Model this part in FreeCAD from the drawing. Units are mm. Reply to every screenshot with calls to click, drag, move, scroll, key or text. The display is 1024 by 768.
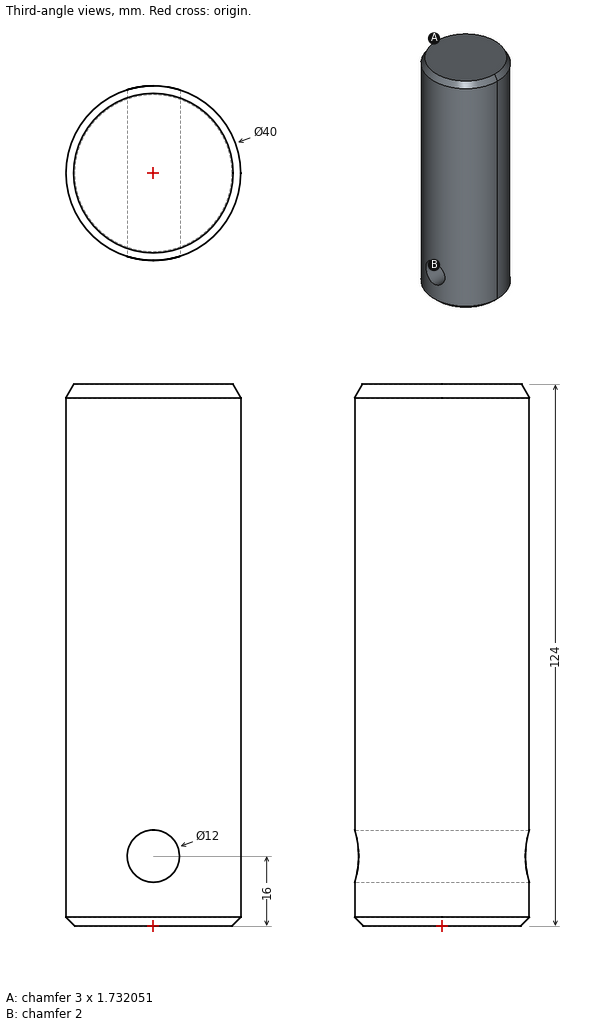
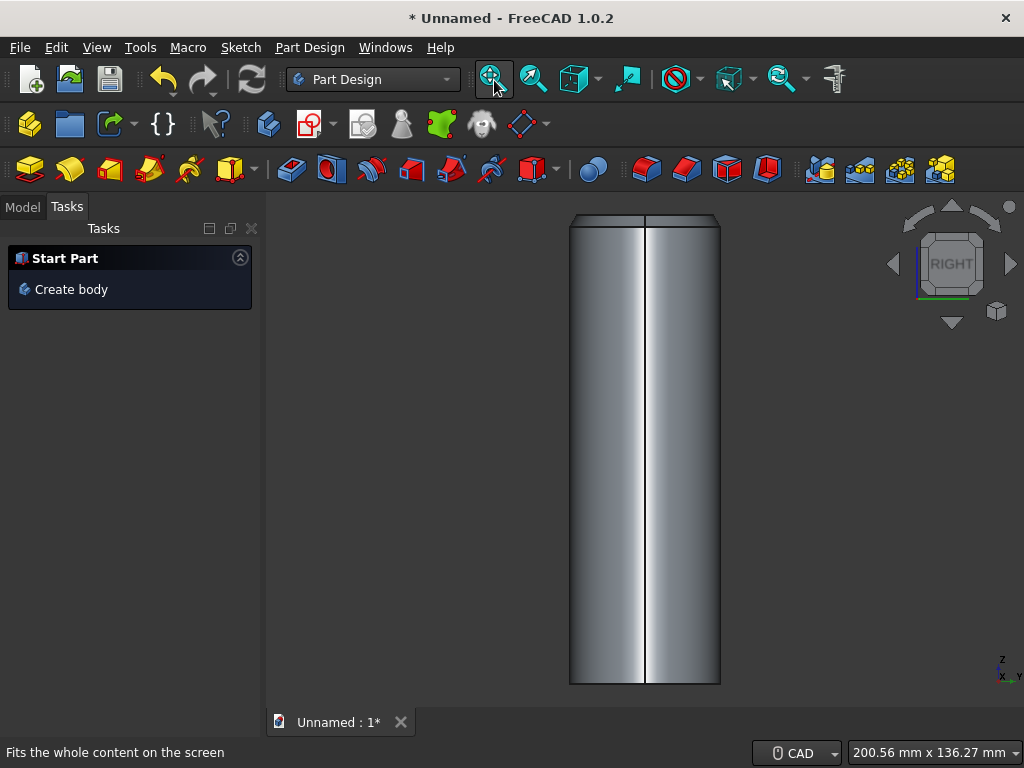
key(5)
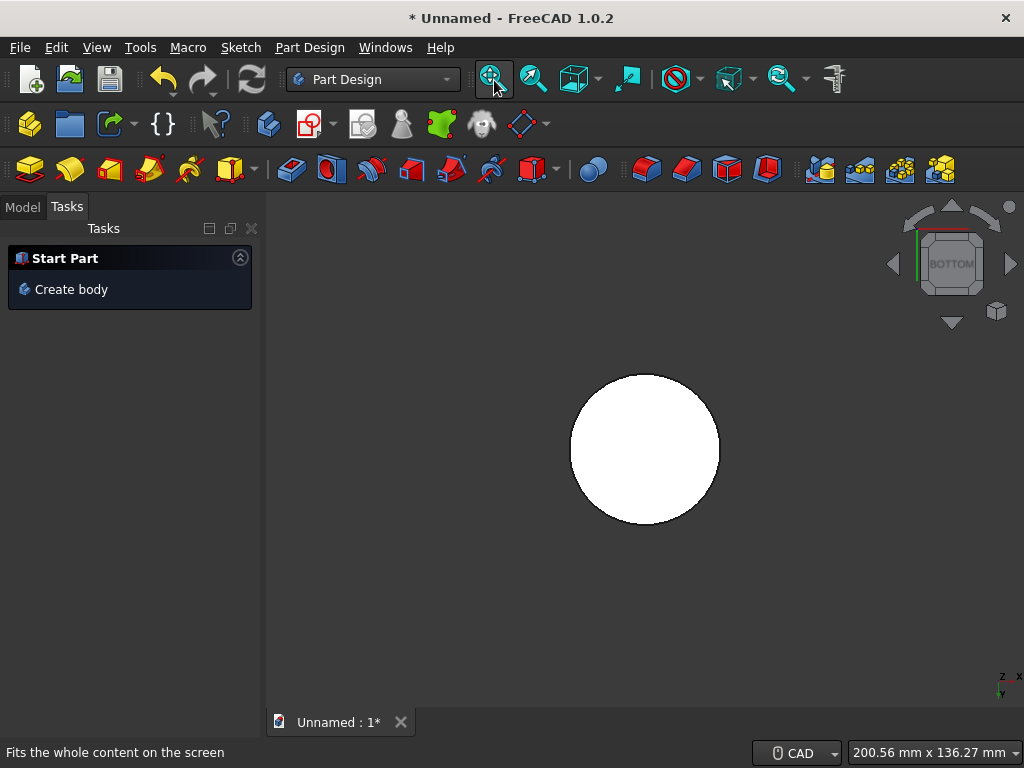
click(494, 80)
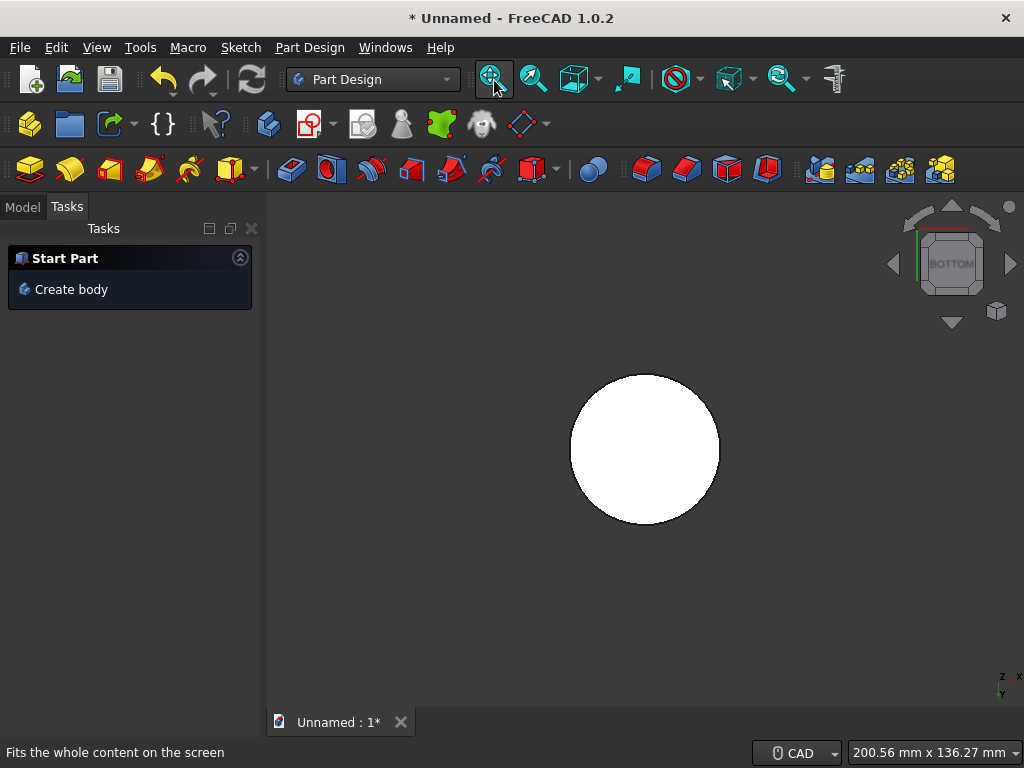
click(569, 448)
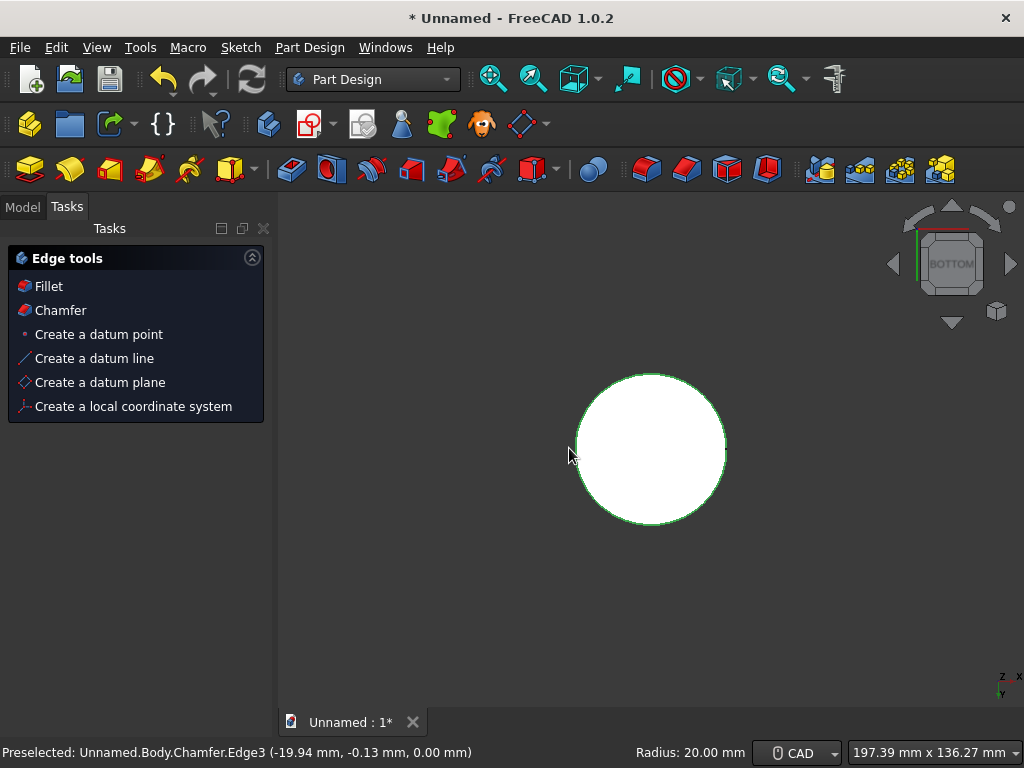
click(688, 170)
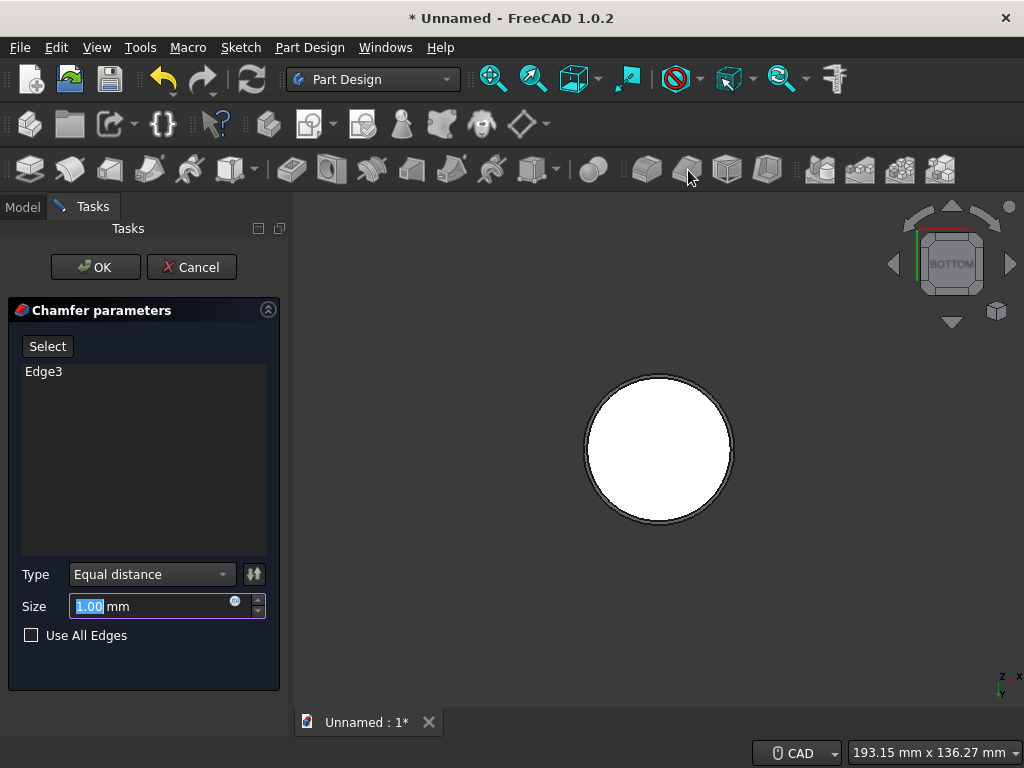
text(2)
key(Tab)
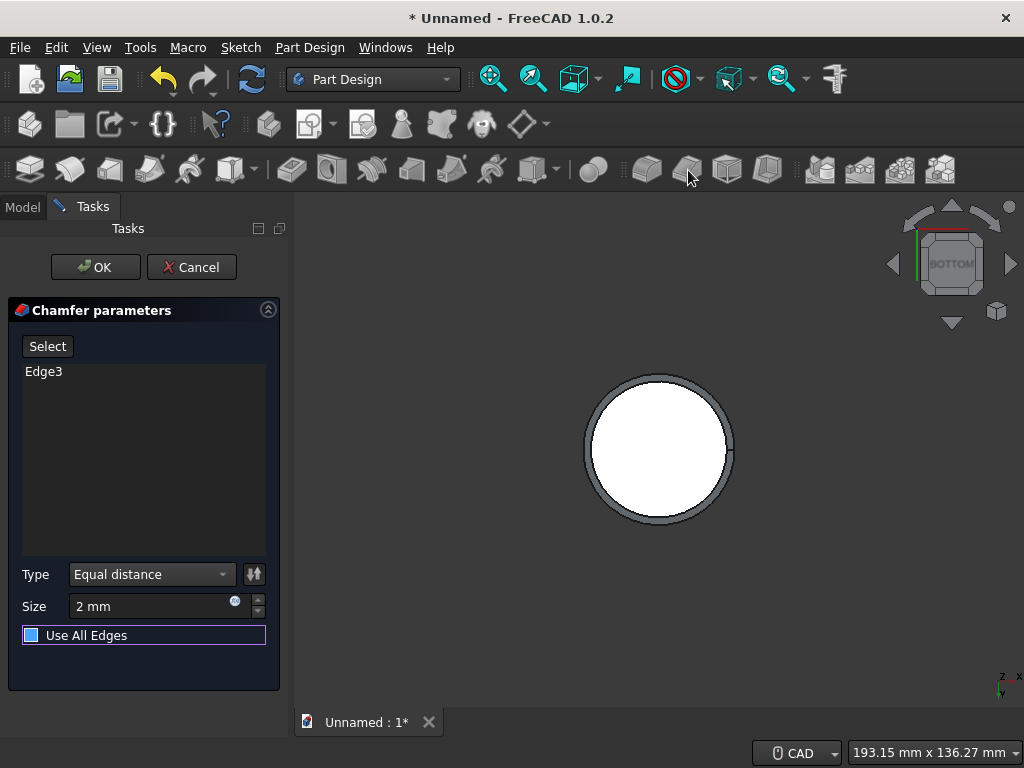
click(96, 267)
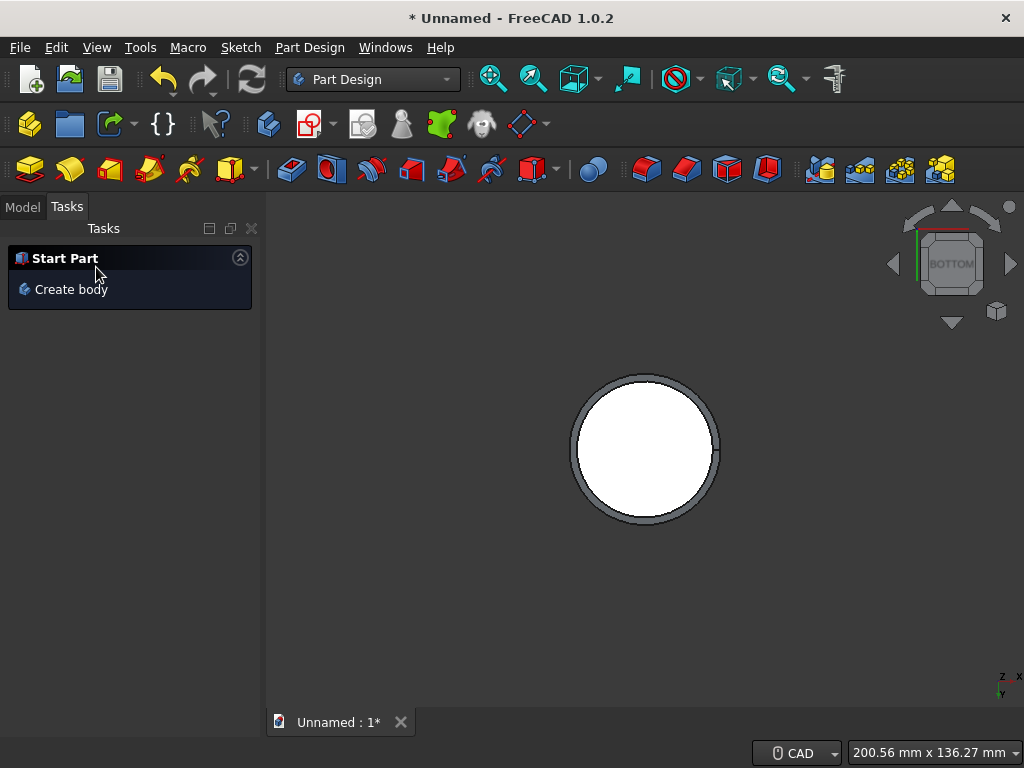
click(494, 80)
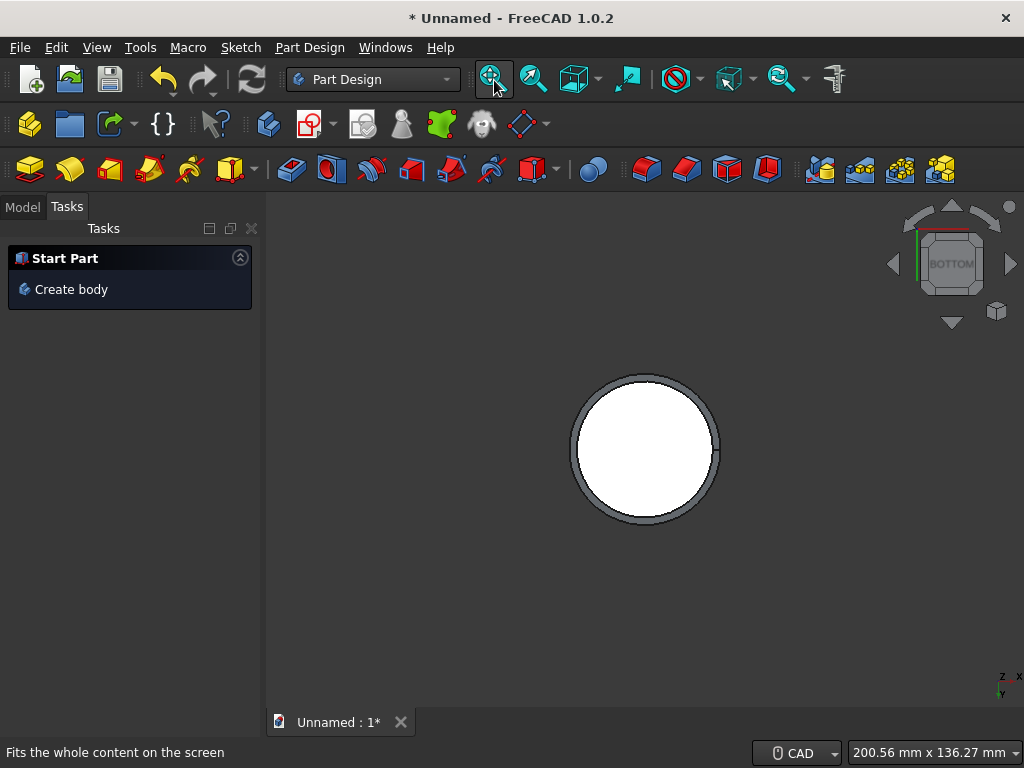
click(310, 124)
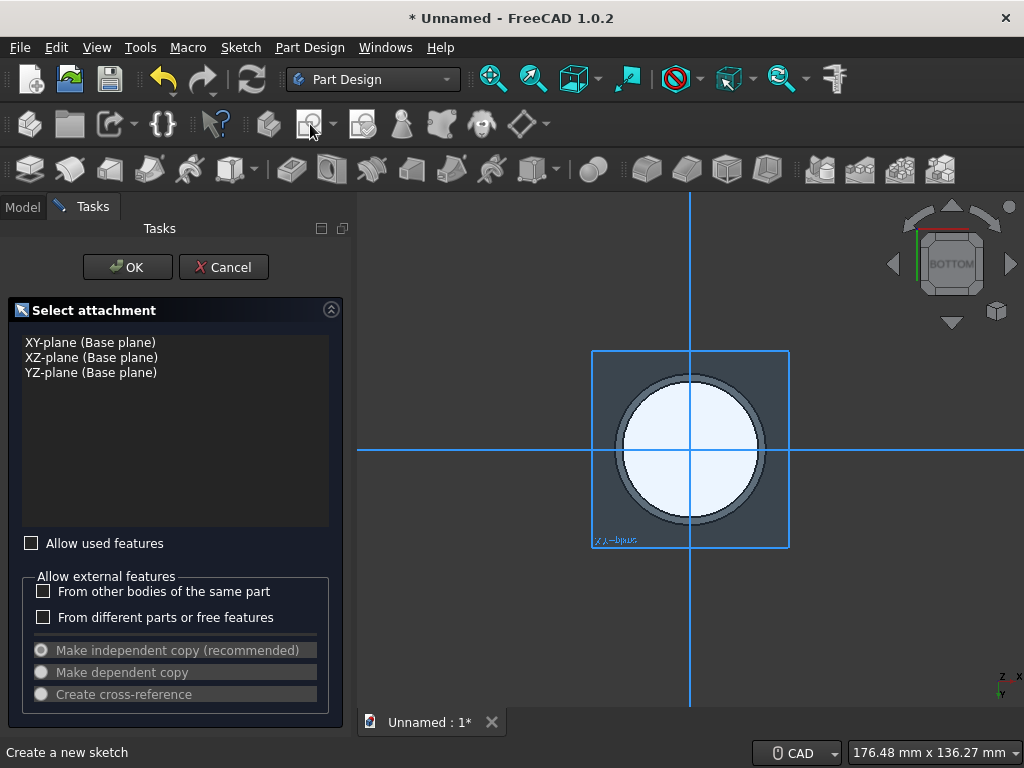
click(82, 358)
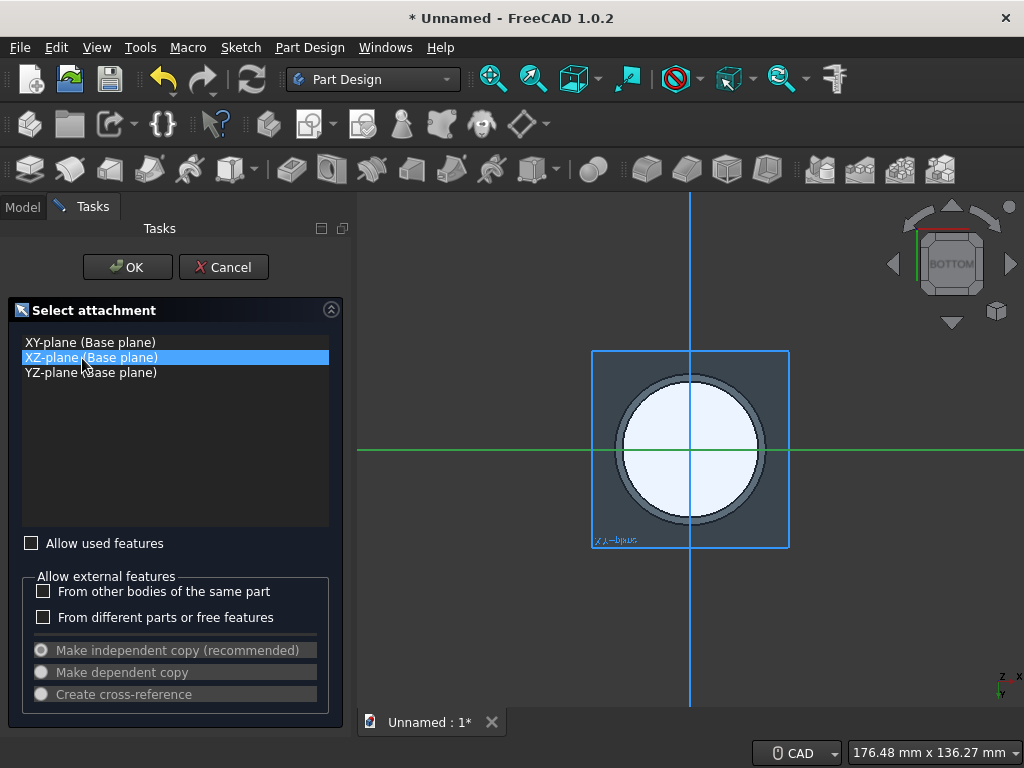
click(128, 267)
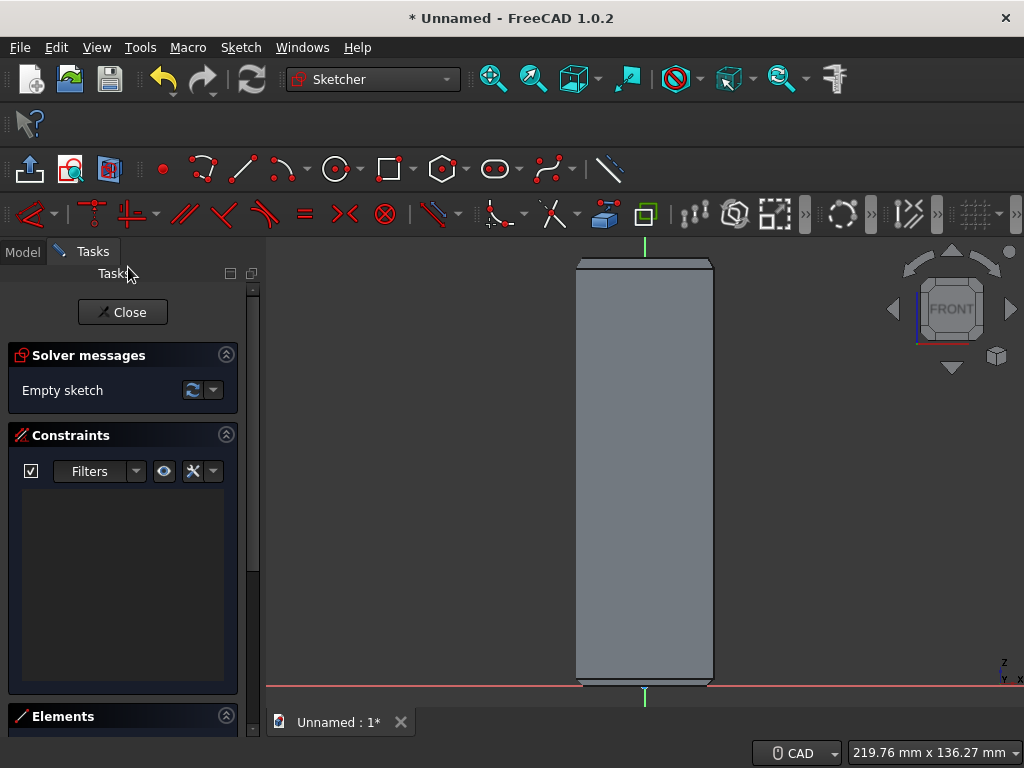
click(110, 170)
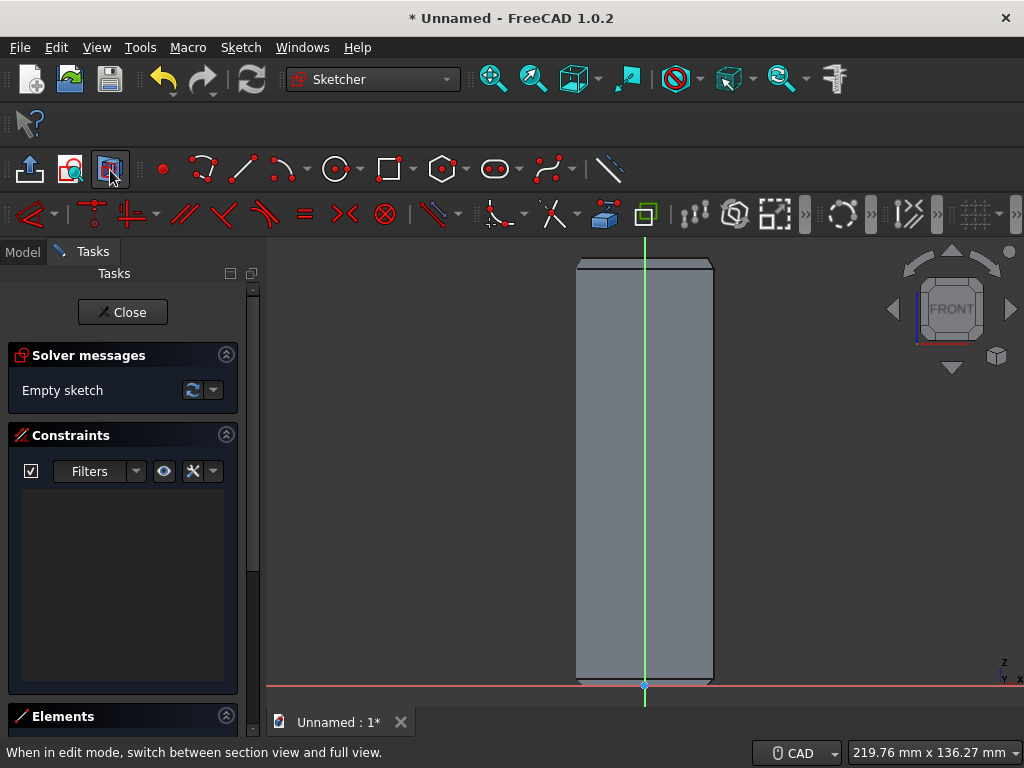
scroll(576, 472, down, 5)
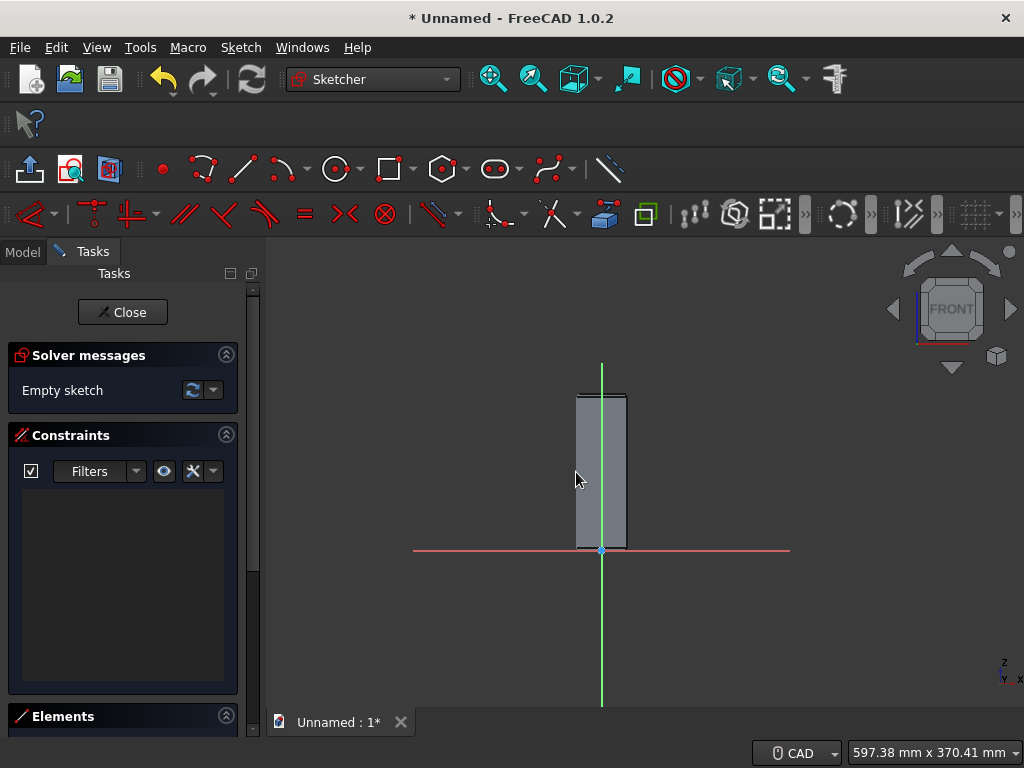
scroll(604, 544, up, 12)